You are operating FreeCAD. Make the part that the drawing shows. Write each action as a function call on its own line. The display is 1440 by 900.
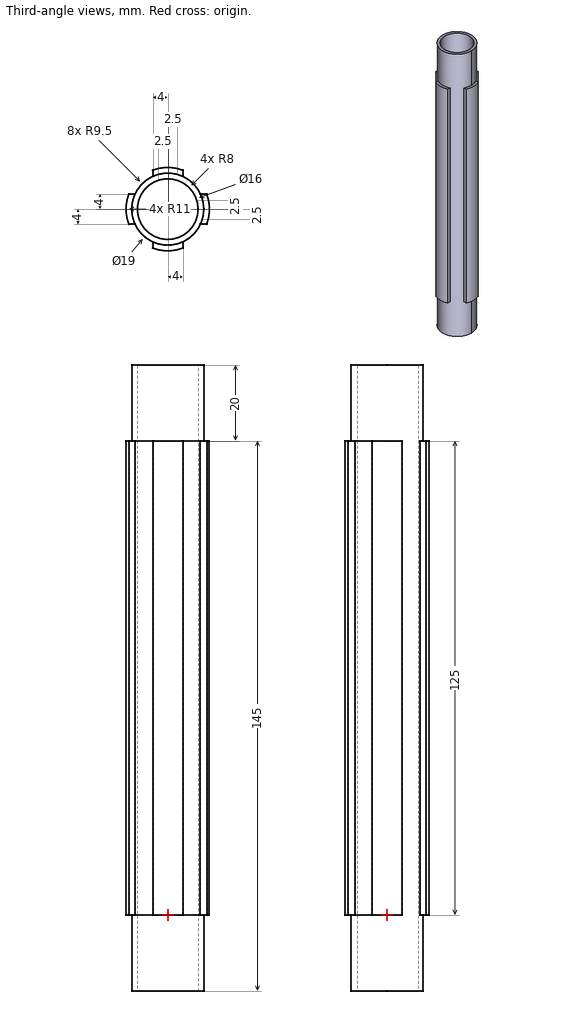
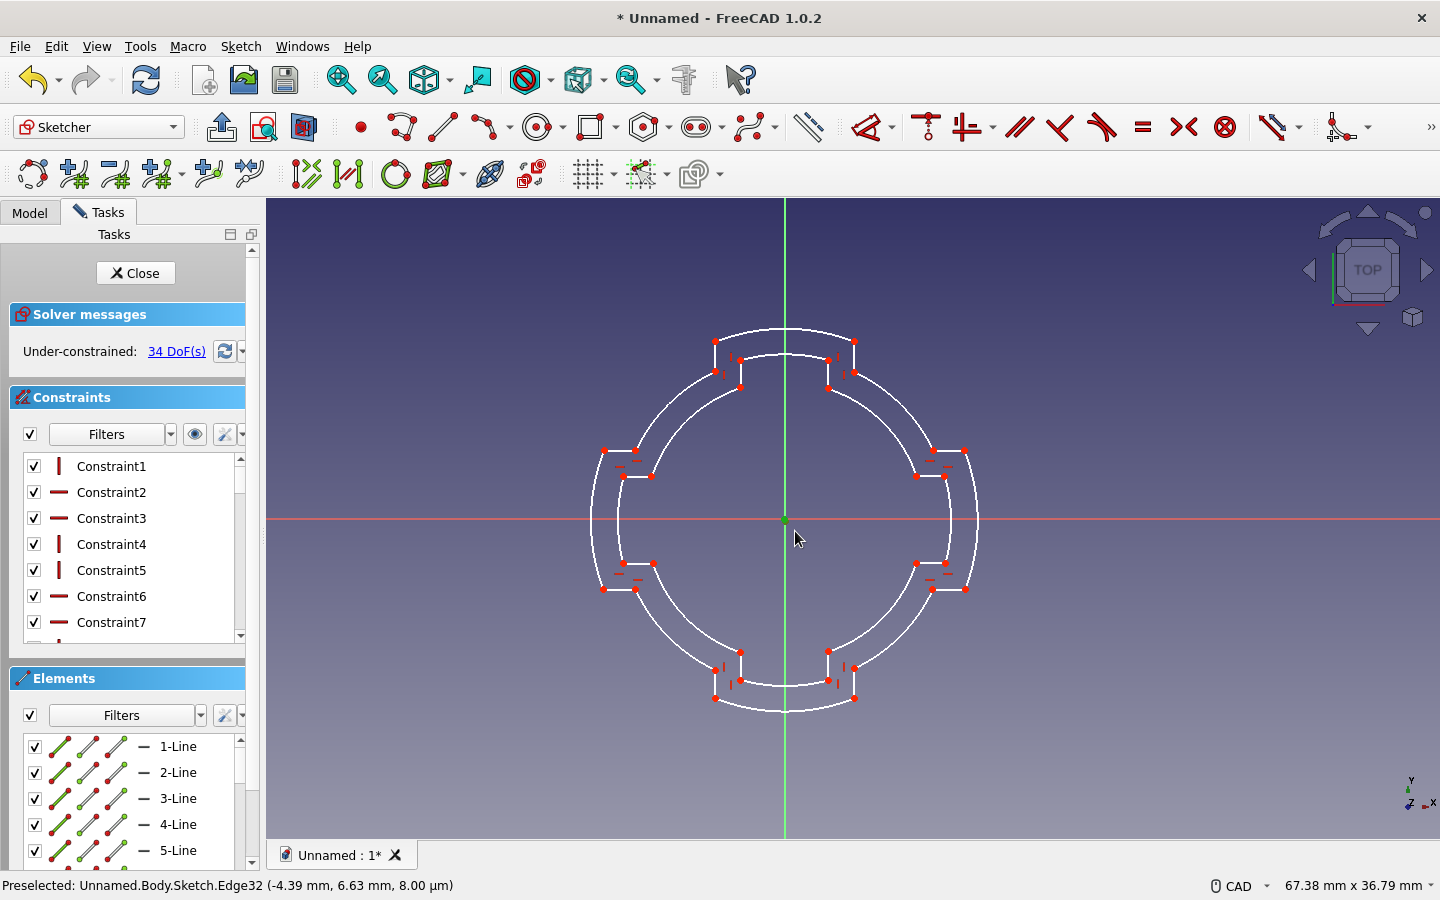
click(926, 128)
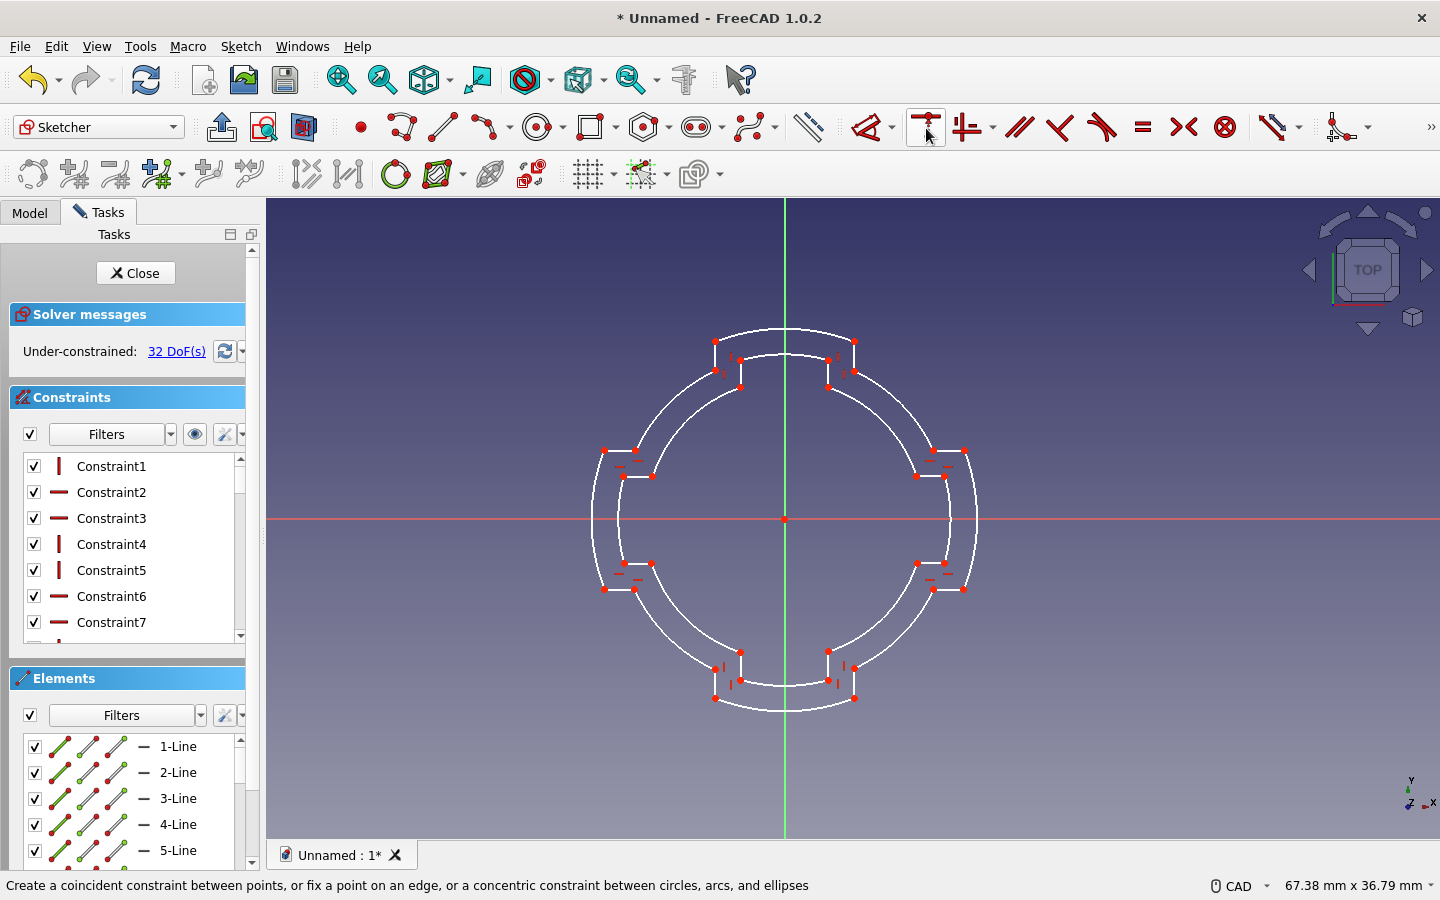
click(686, 389)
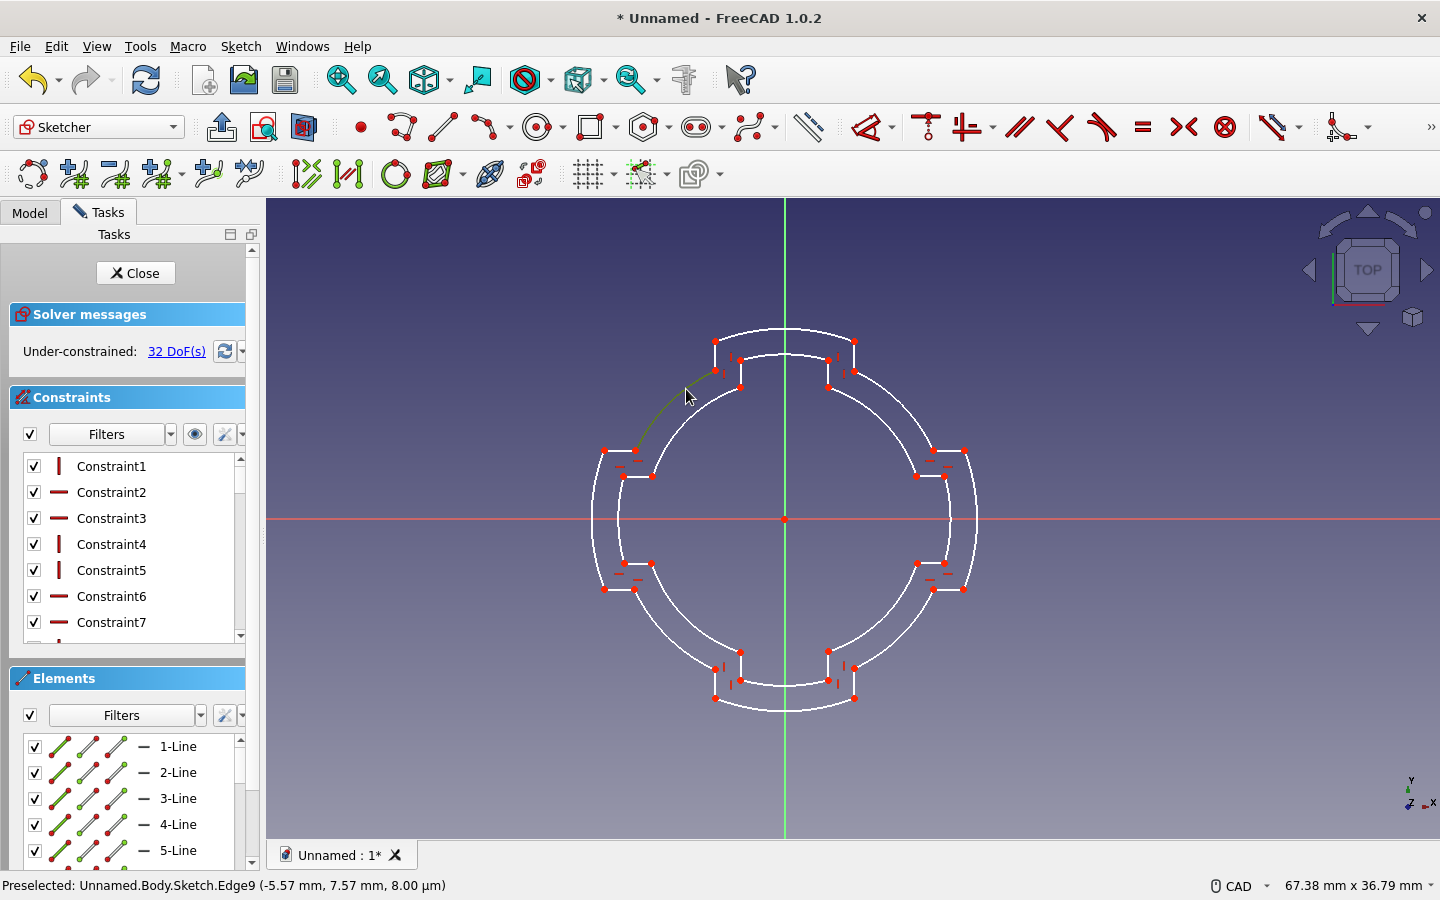
click(653, 620)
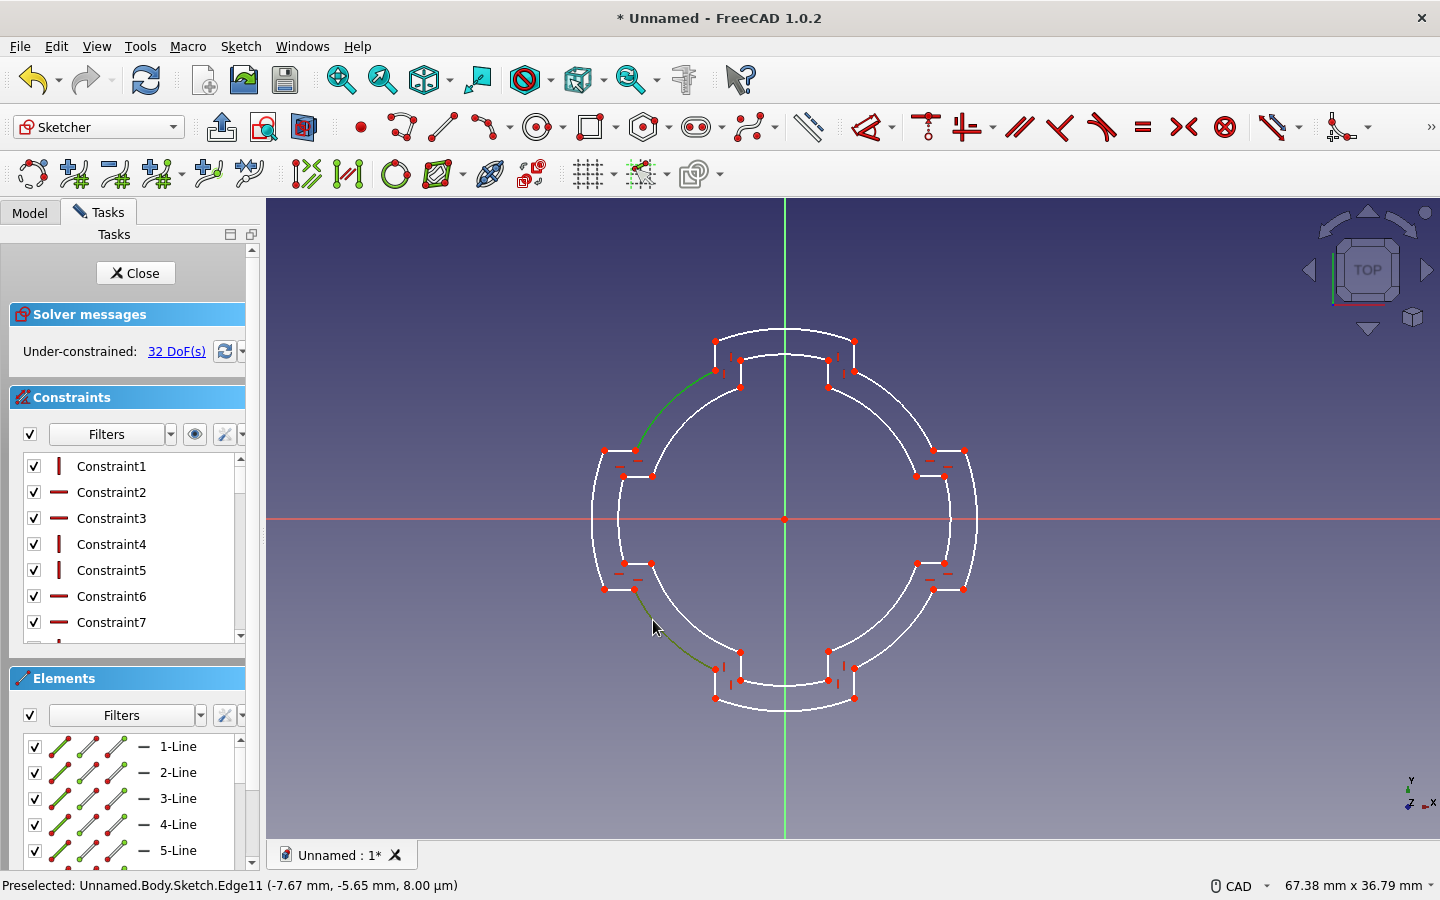
click(884, 651)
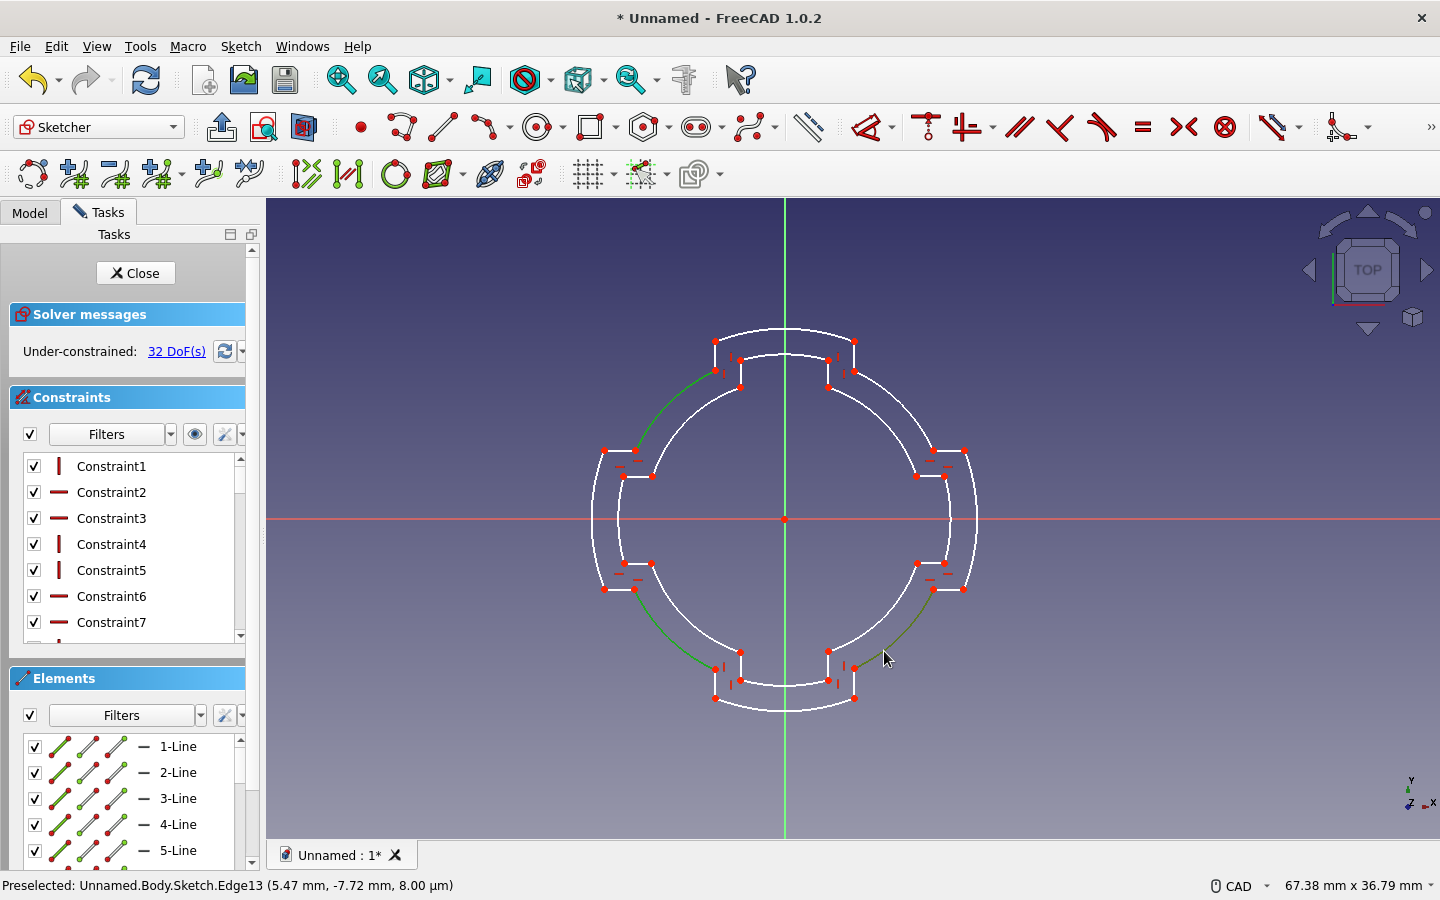
click(916, 421)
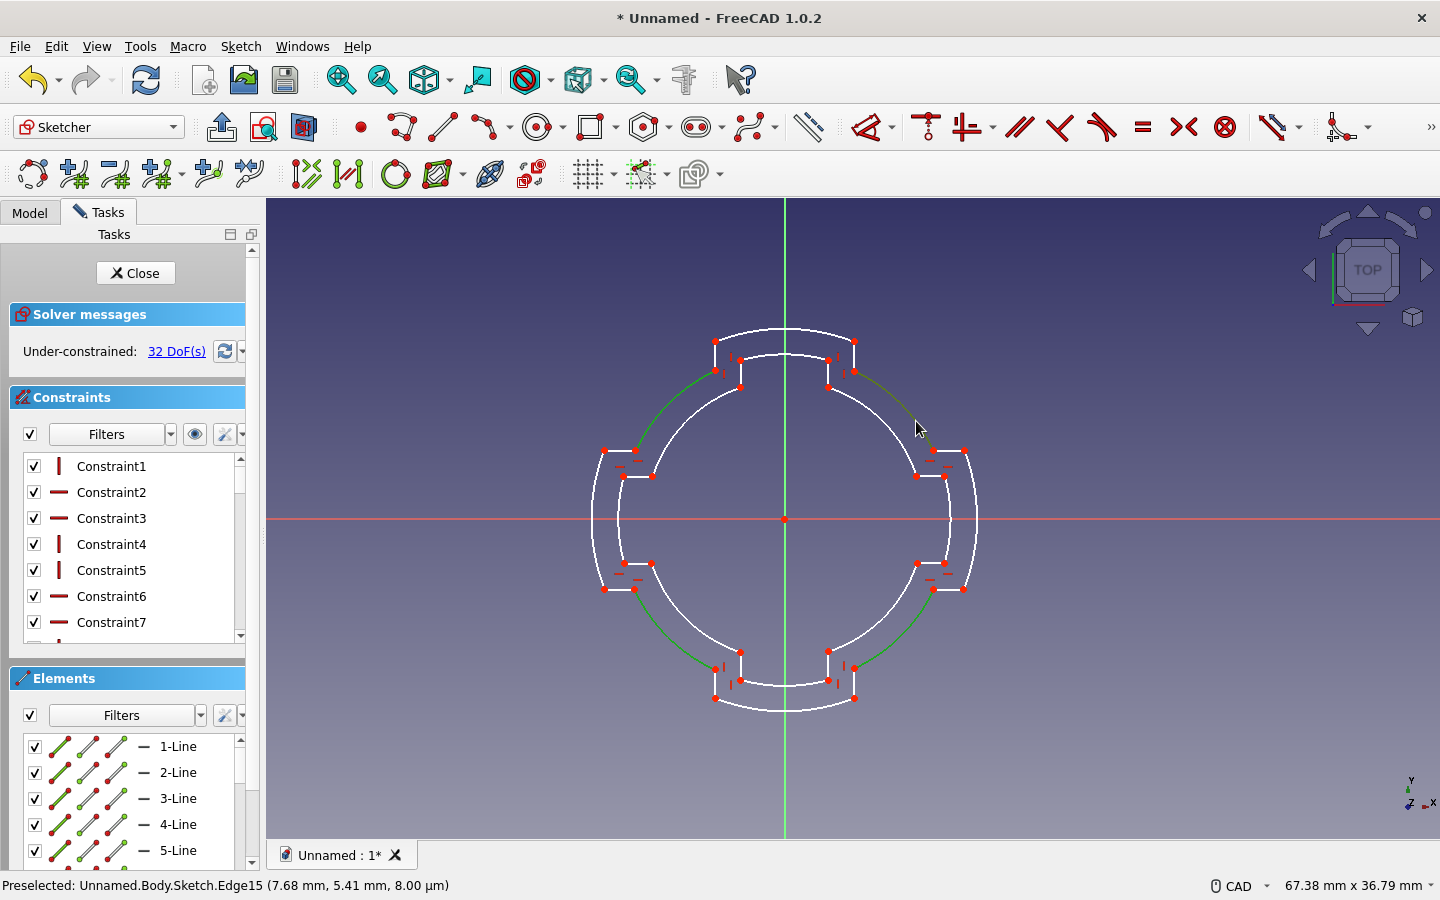
click(802, 355)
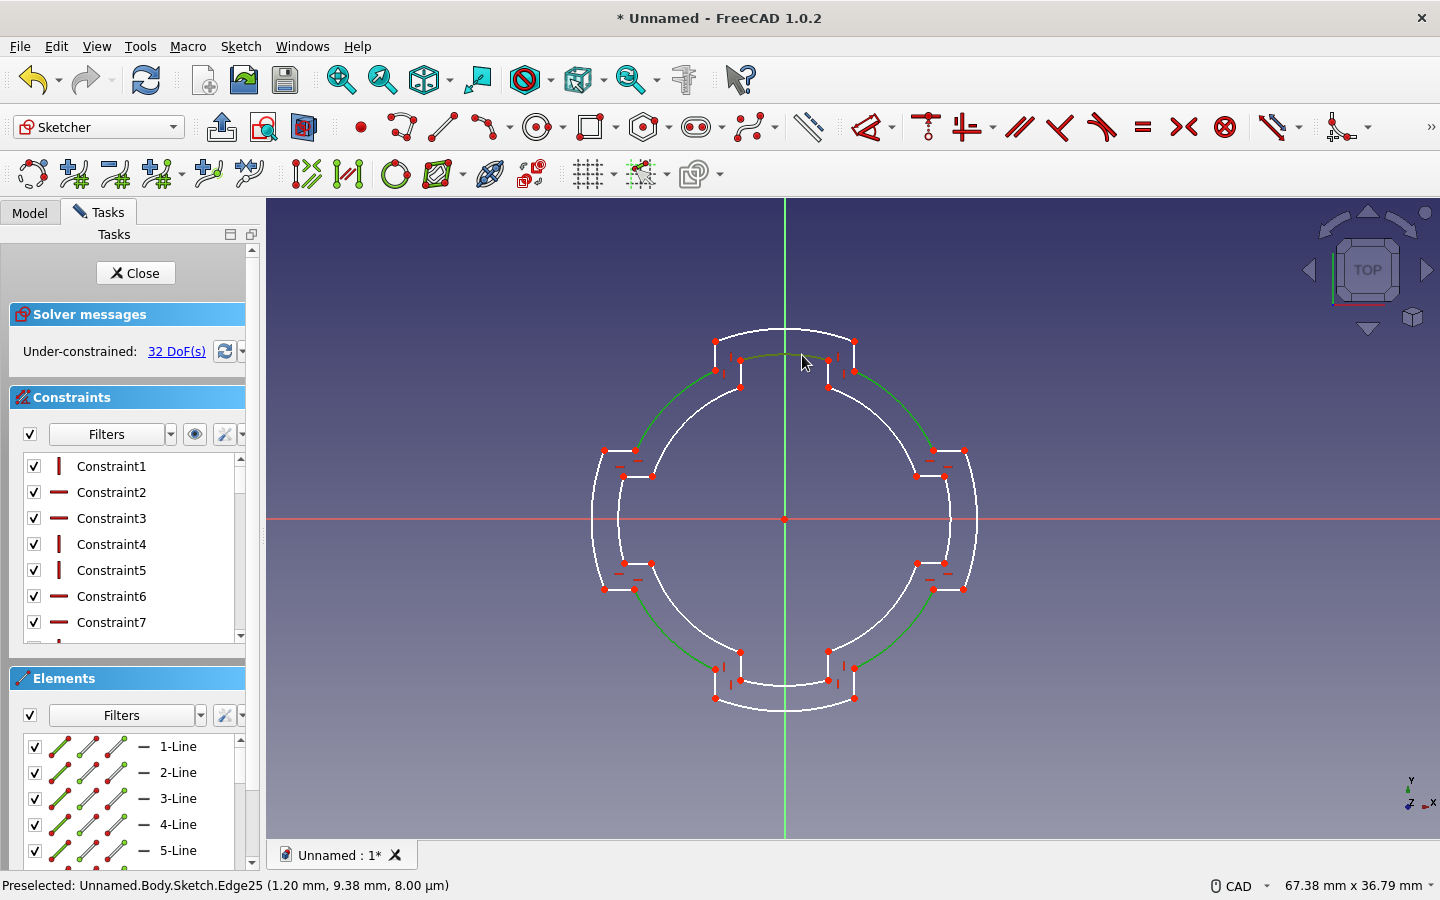
click(950, 537)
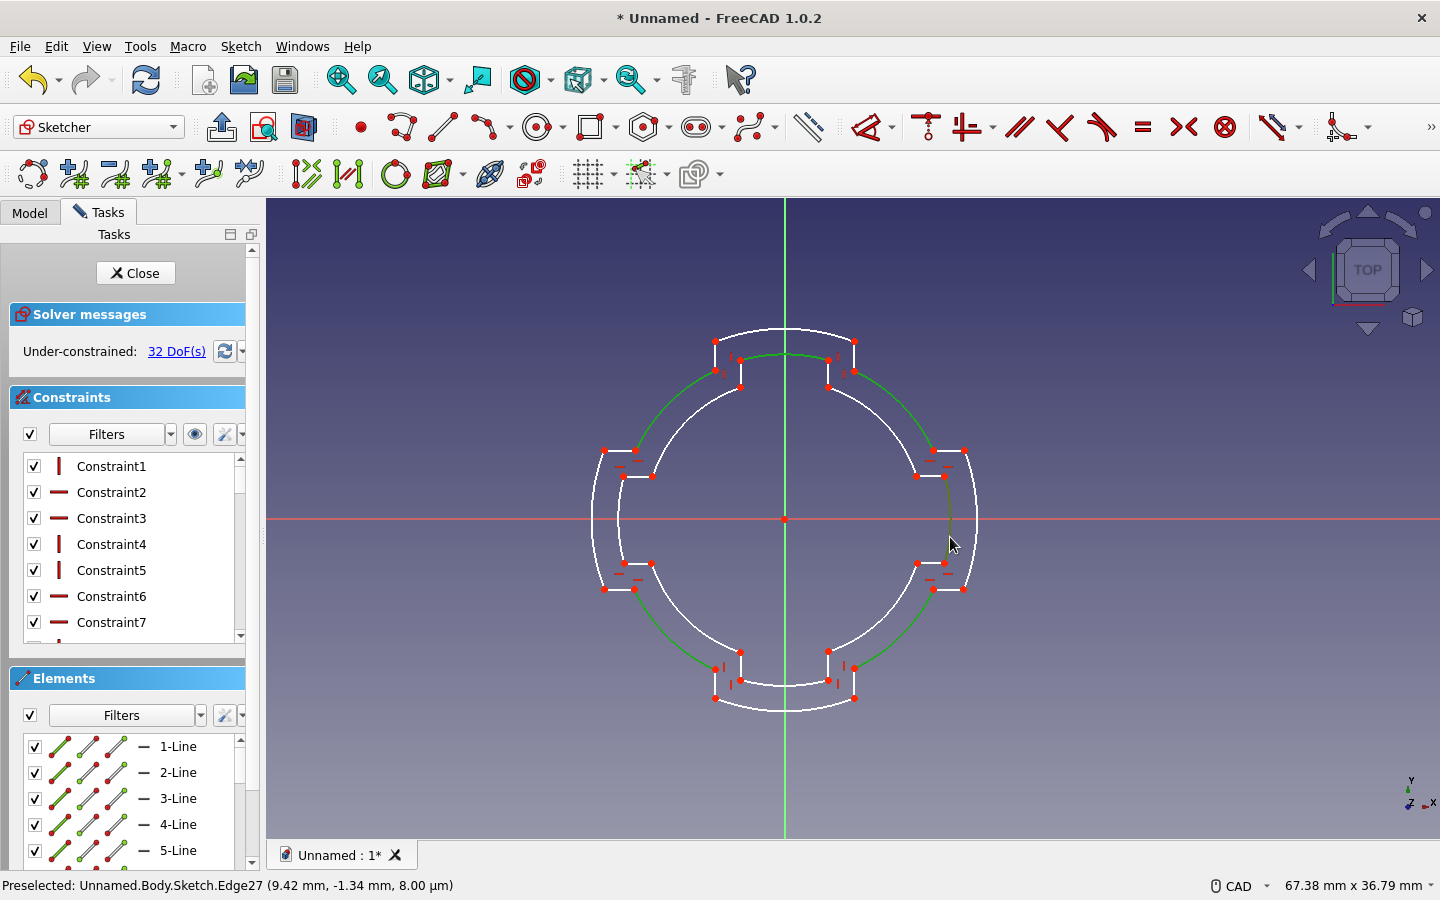
click(767, 685)